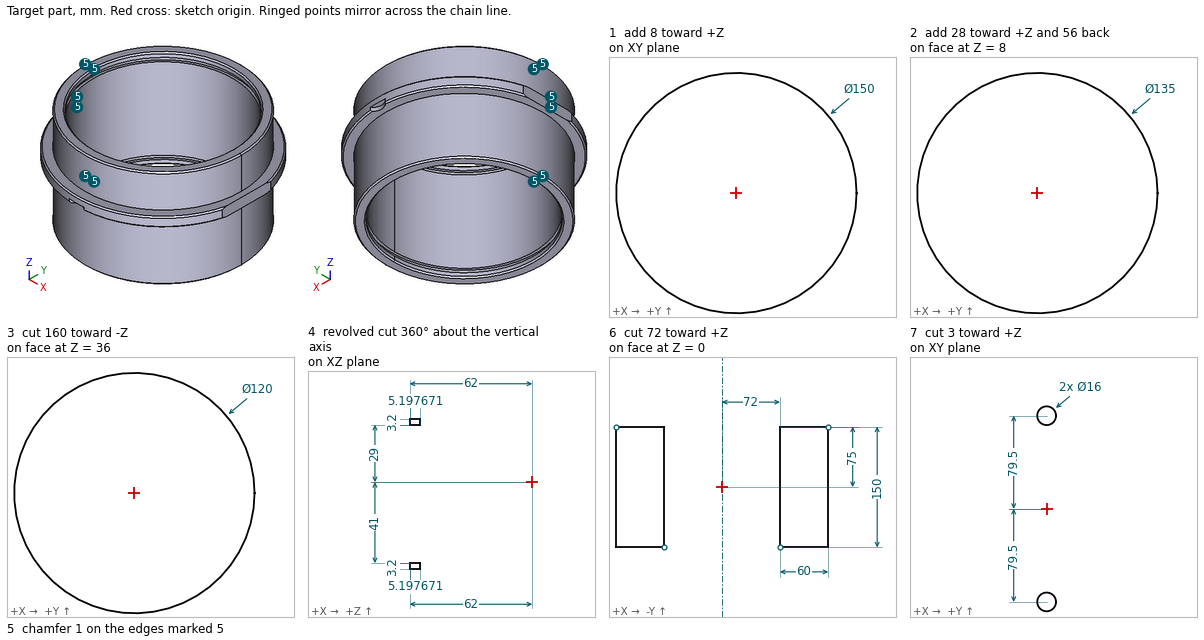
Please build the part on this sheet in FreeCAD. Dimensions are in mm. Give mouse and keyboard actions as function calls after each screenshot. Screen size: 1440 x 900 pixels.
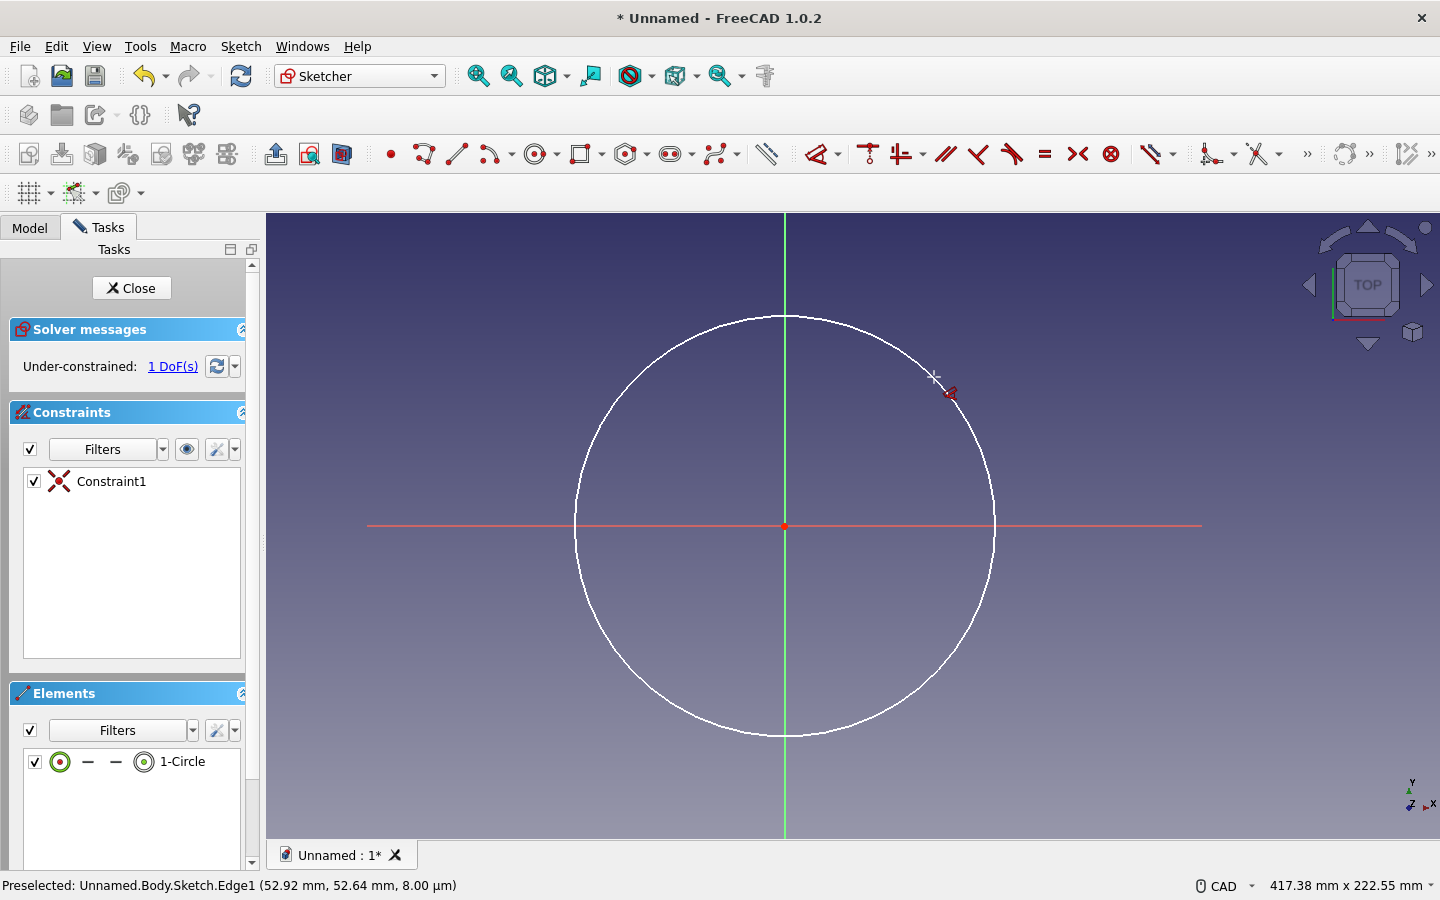
click(933, 377)
click(956, 354)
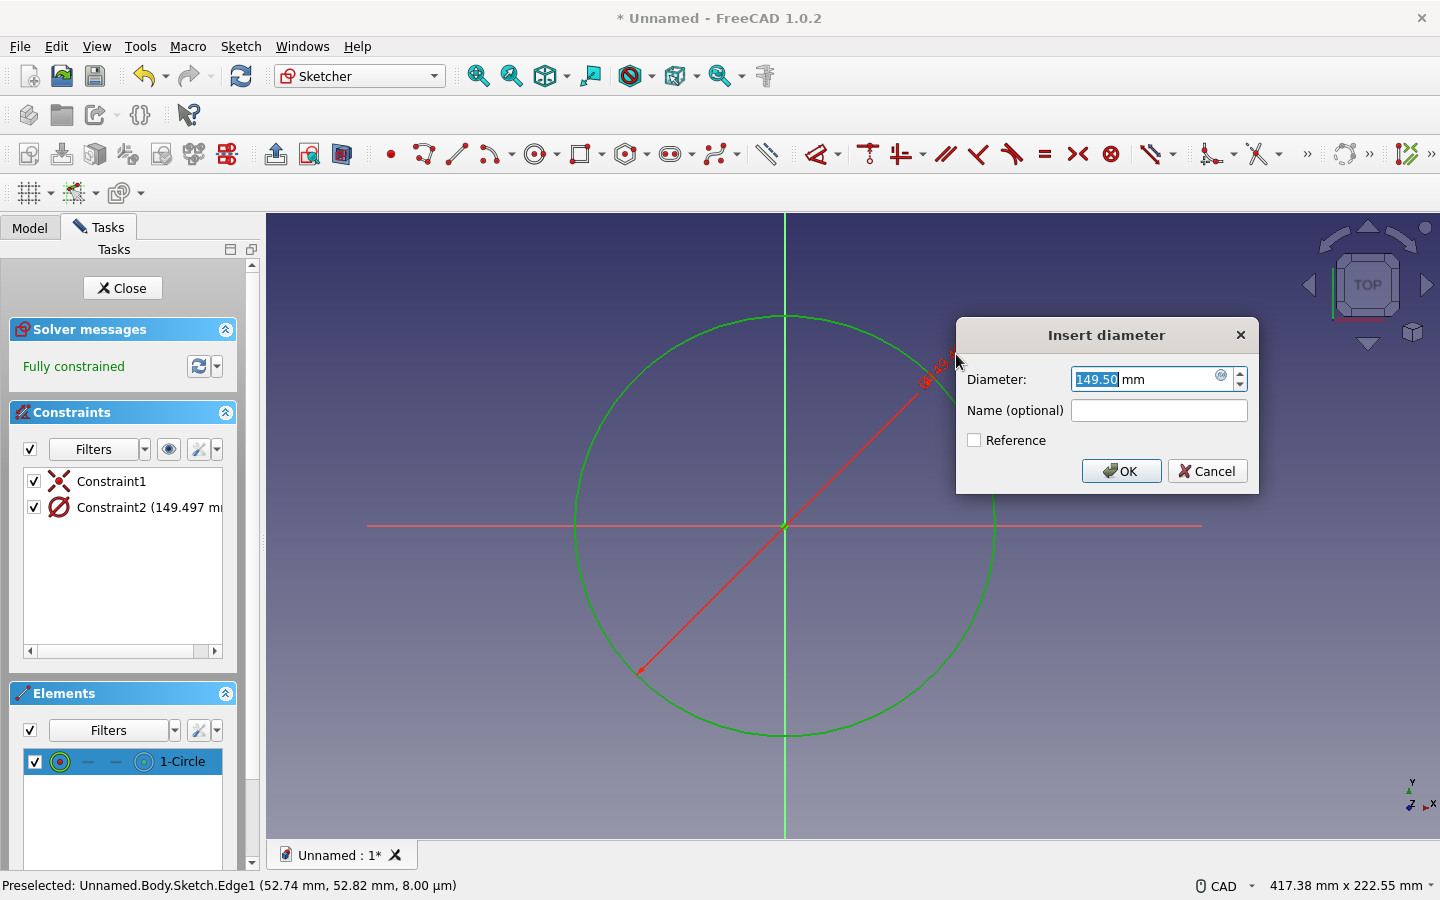
text(150)
key(Return)
key(Escape)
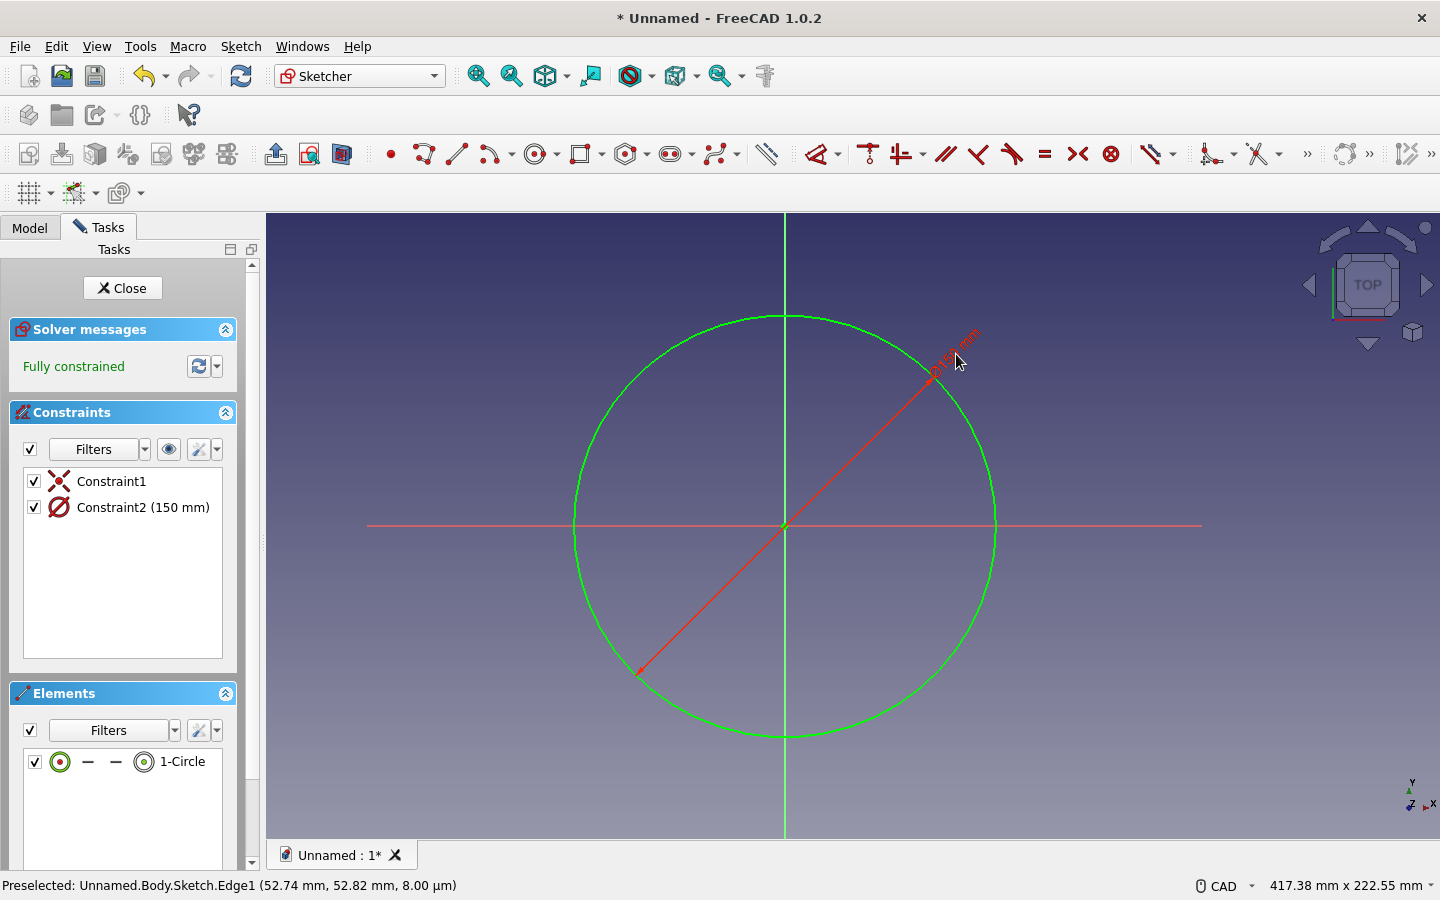
click(123, 288)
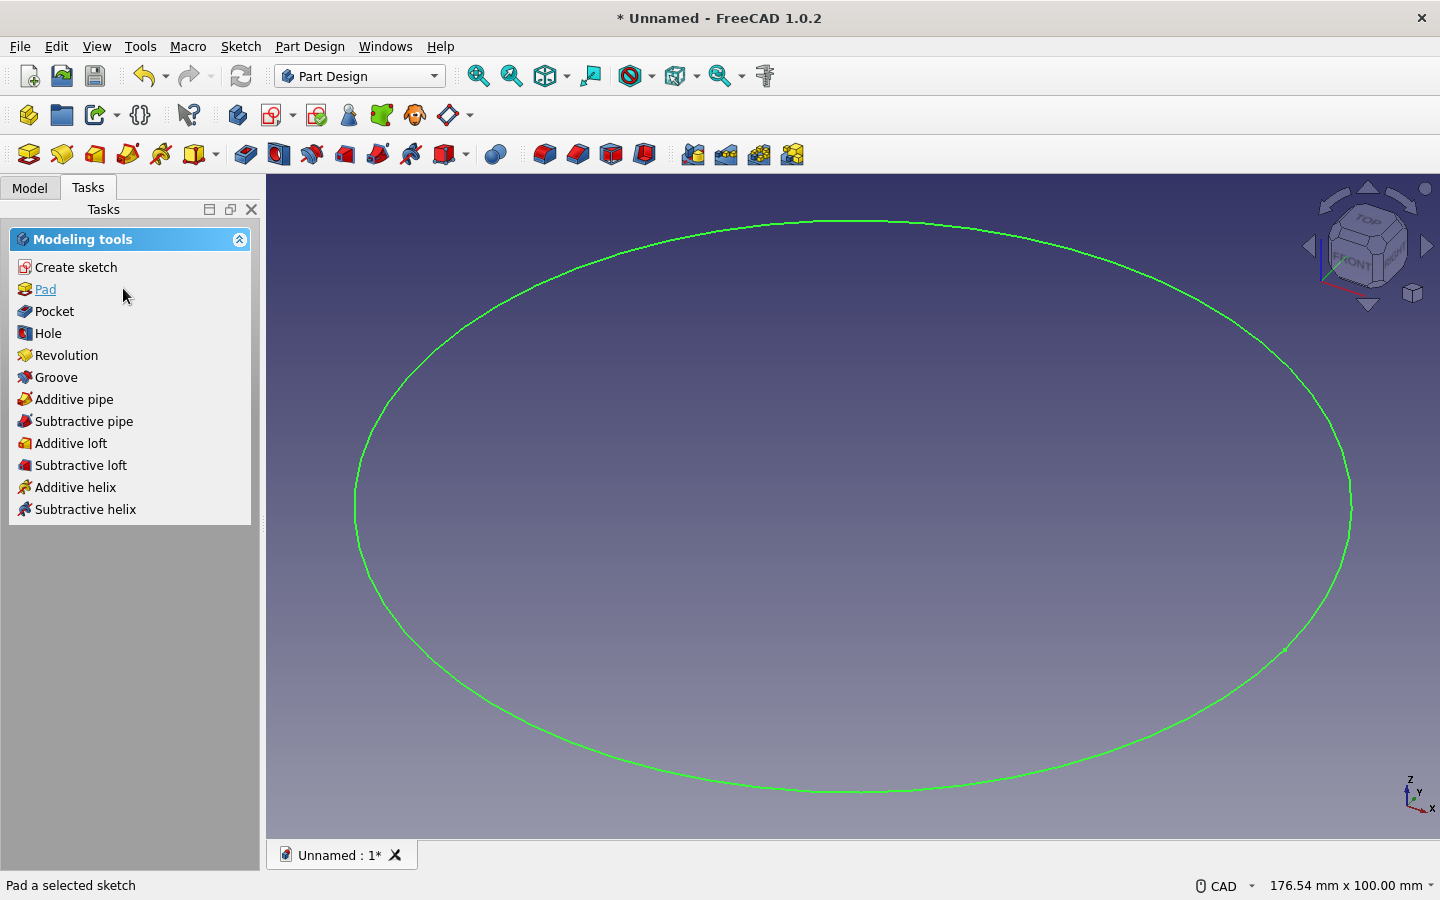
click(29, 154)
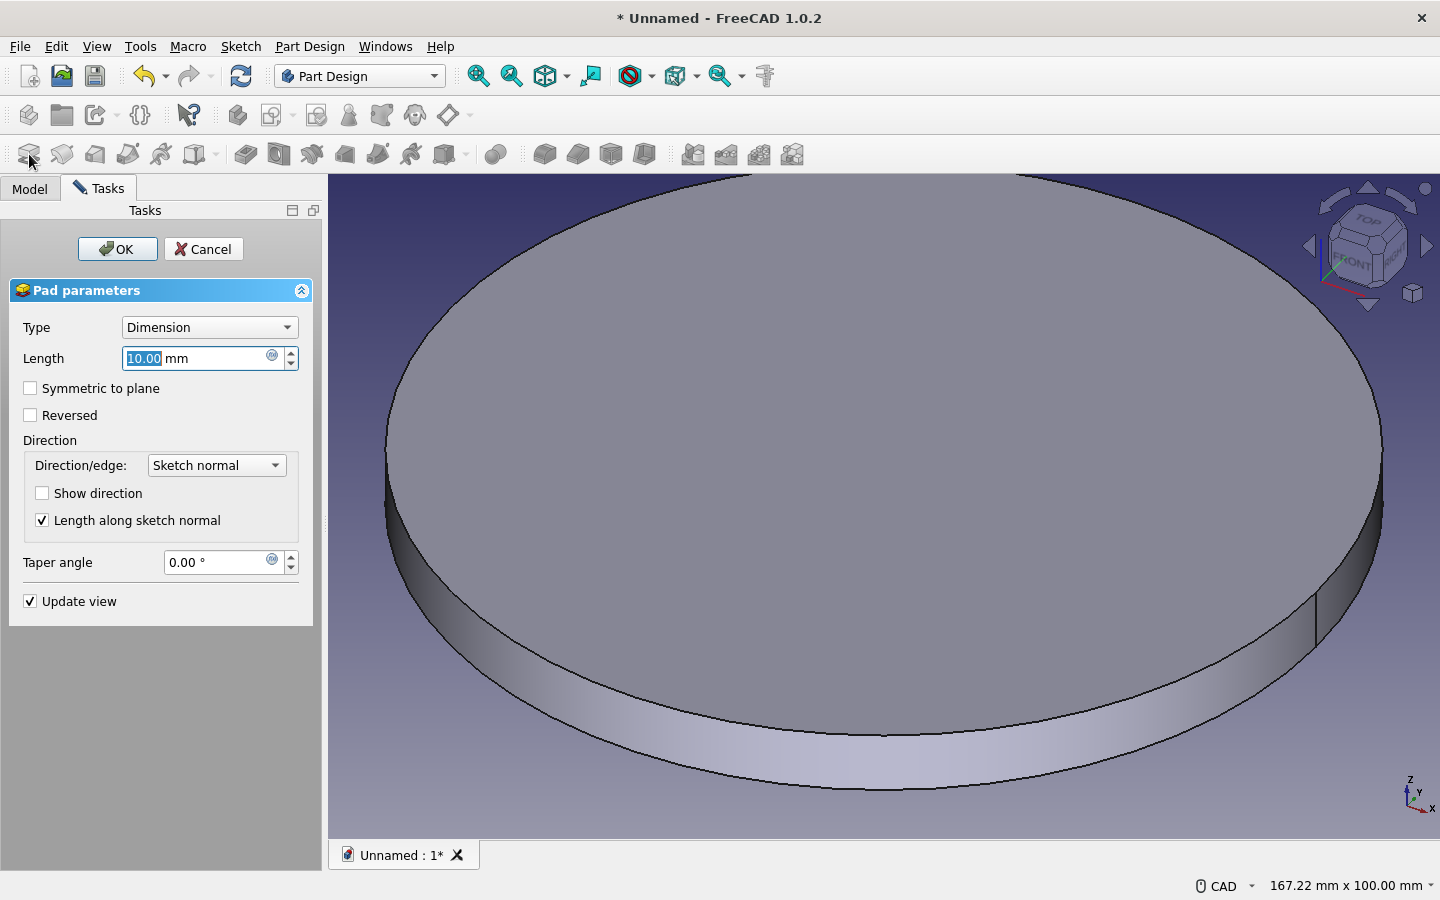
text(8)
key(Tab)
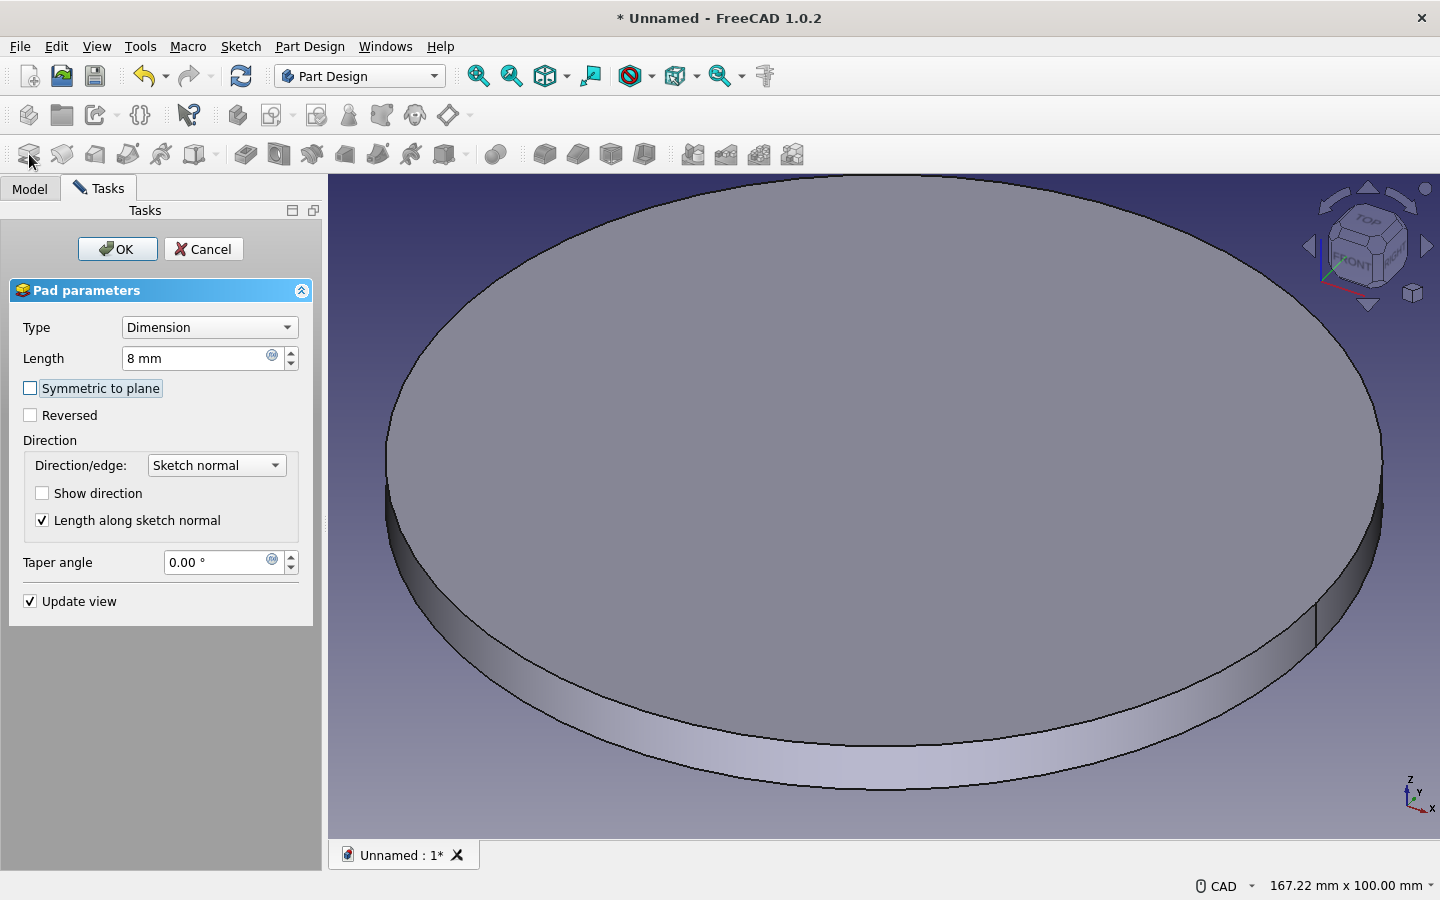
click(118, 249)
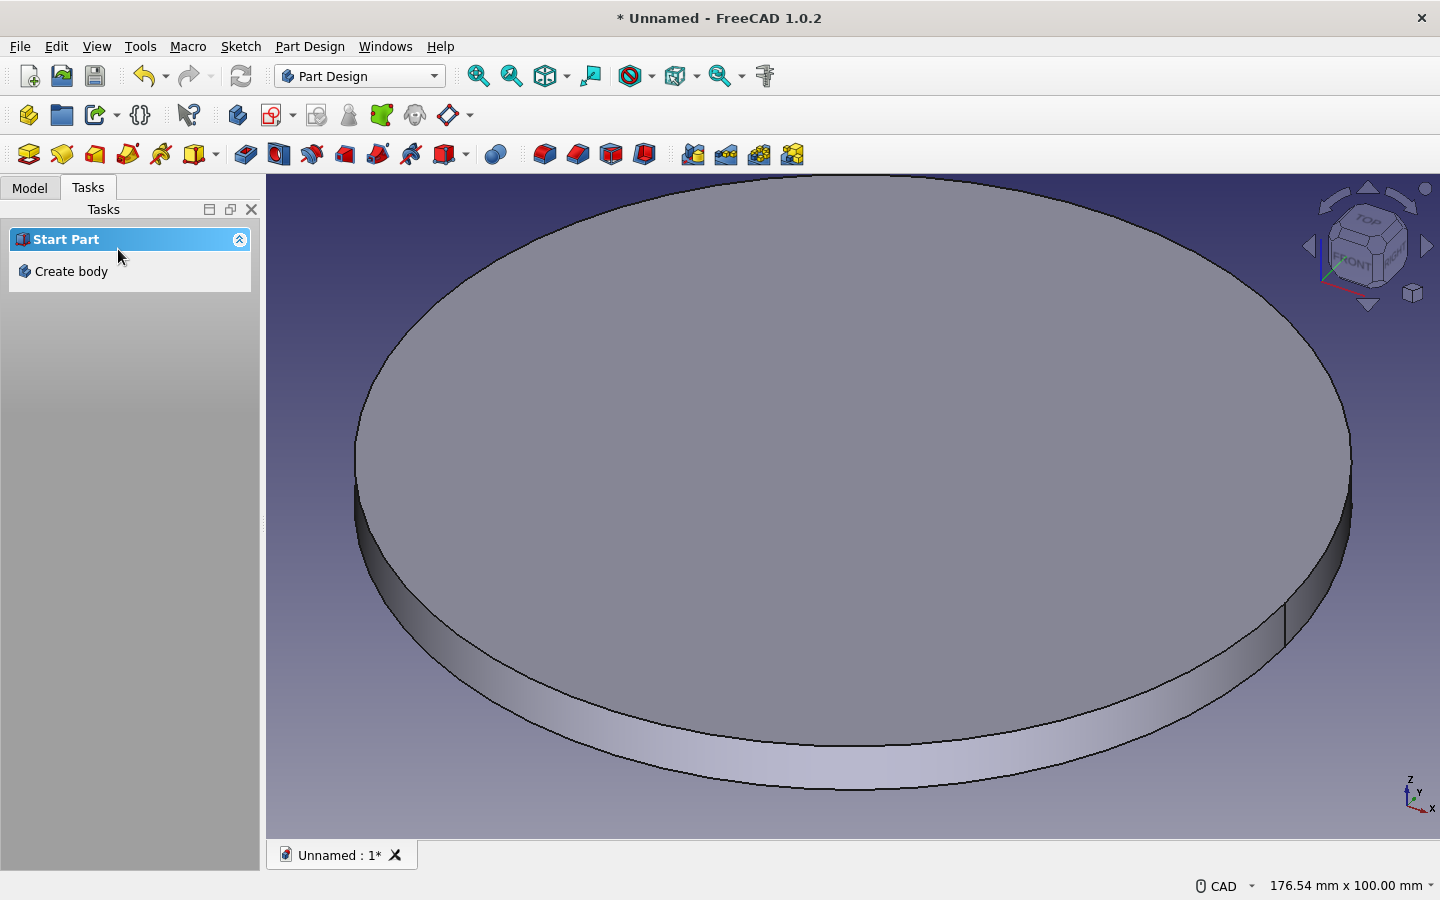
key(v)
key(f)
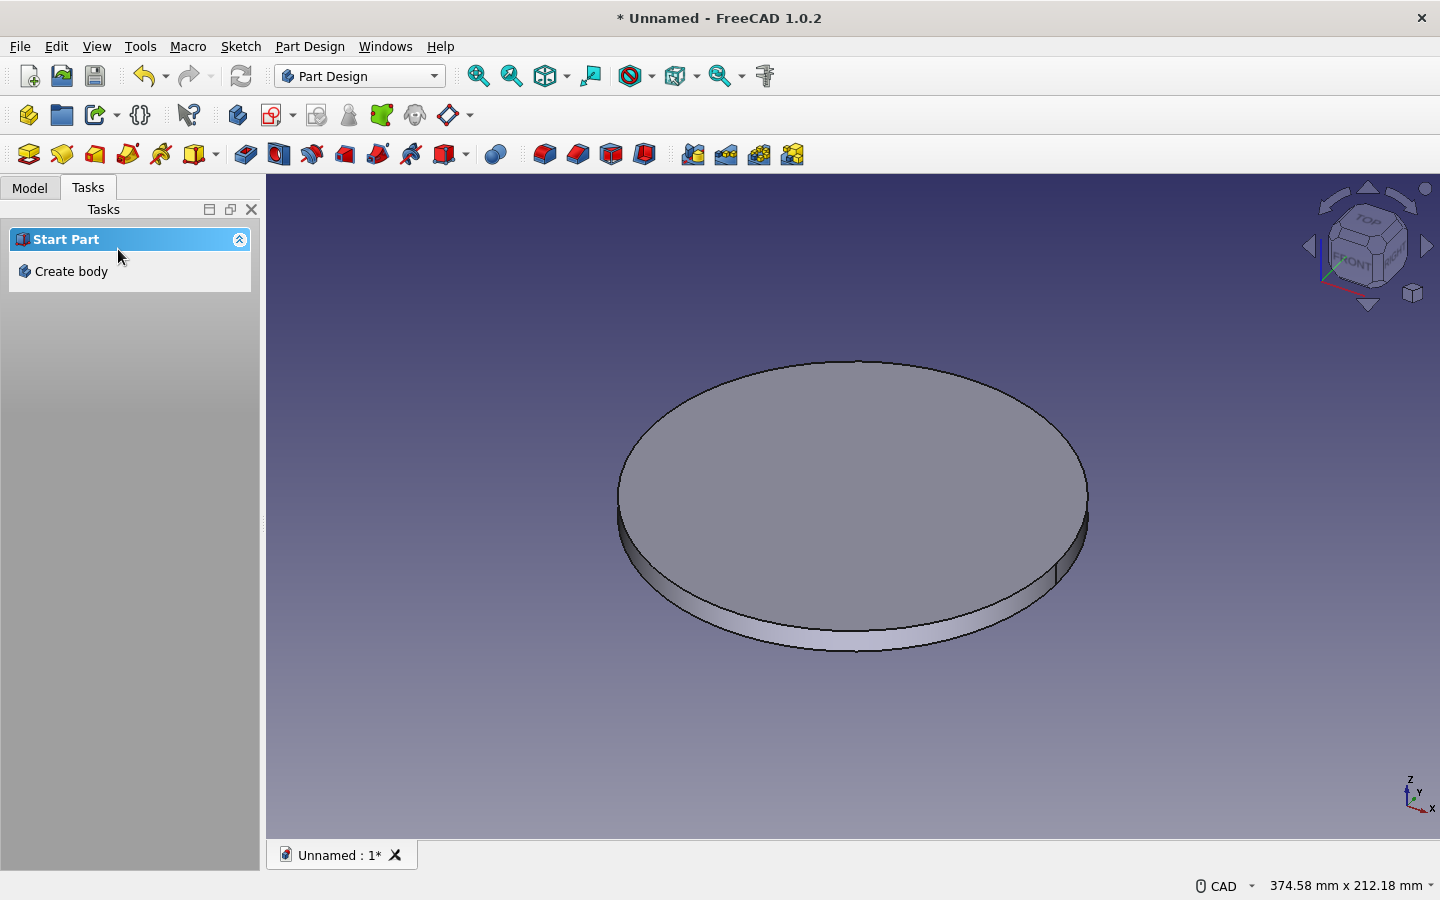
click(853, 495)